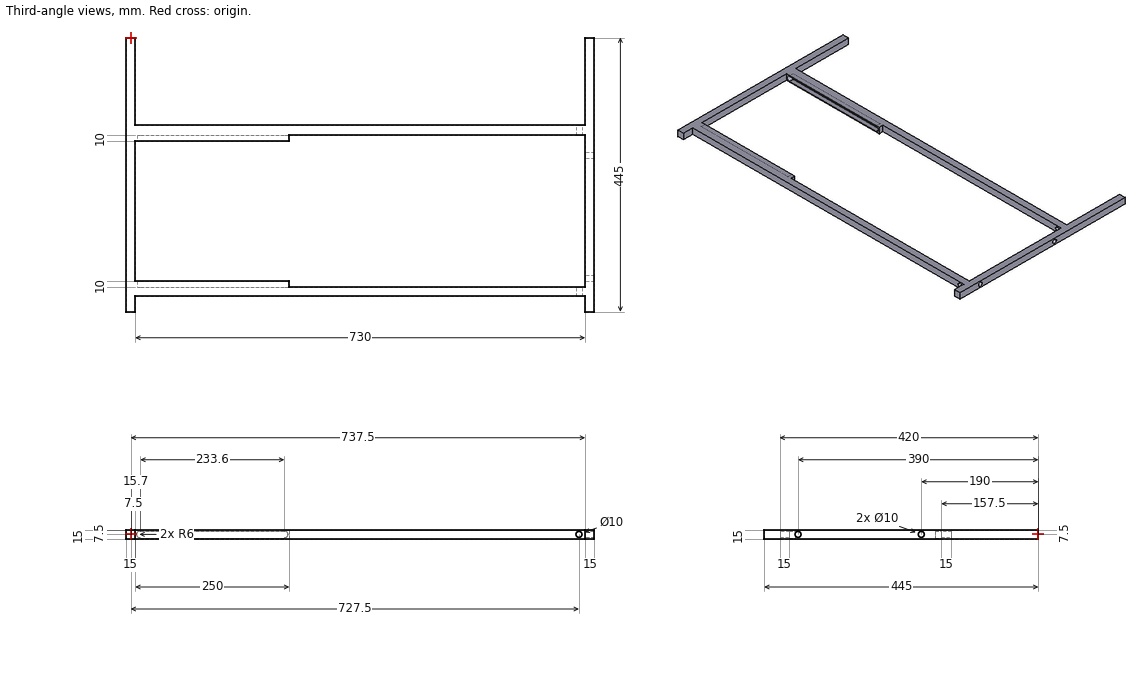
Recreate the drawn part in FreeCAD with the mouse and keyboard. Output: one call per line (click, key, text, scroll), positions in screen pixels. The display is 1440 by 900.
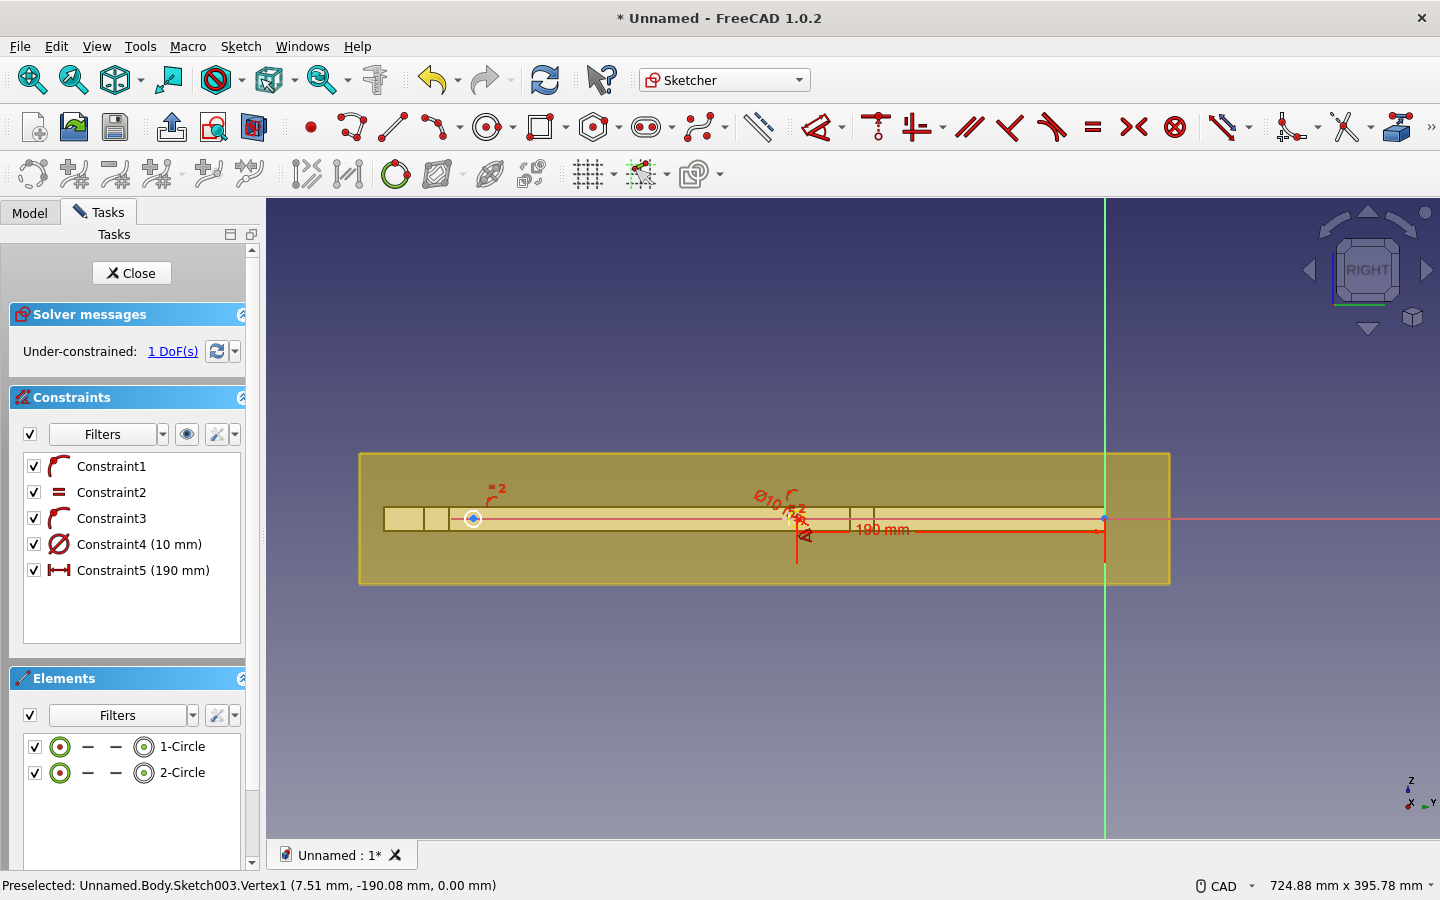
click(473, 519)
click(789, 553)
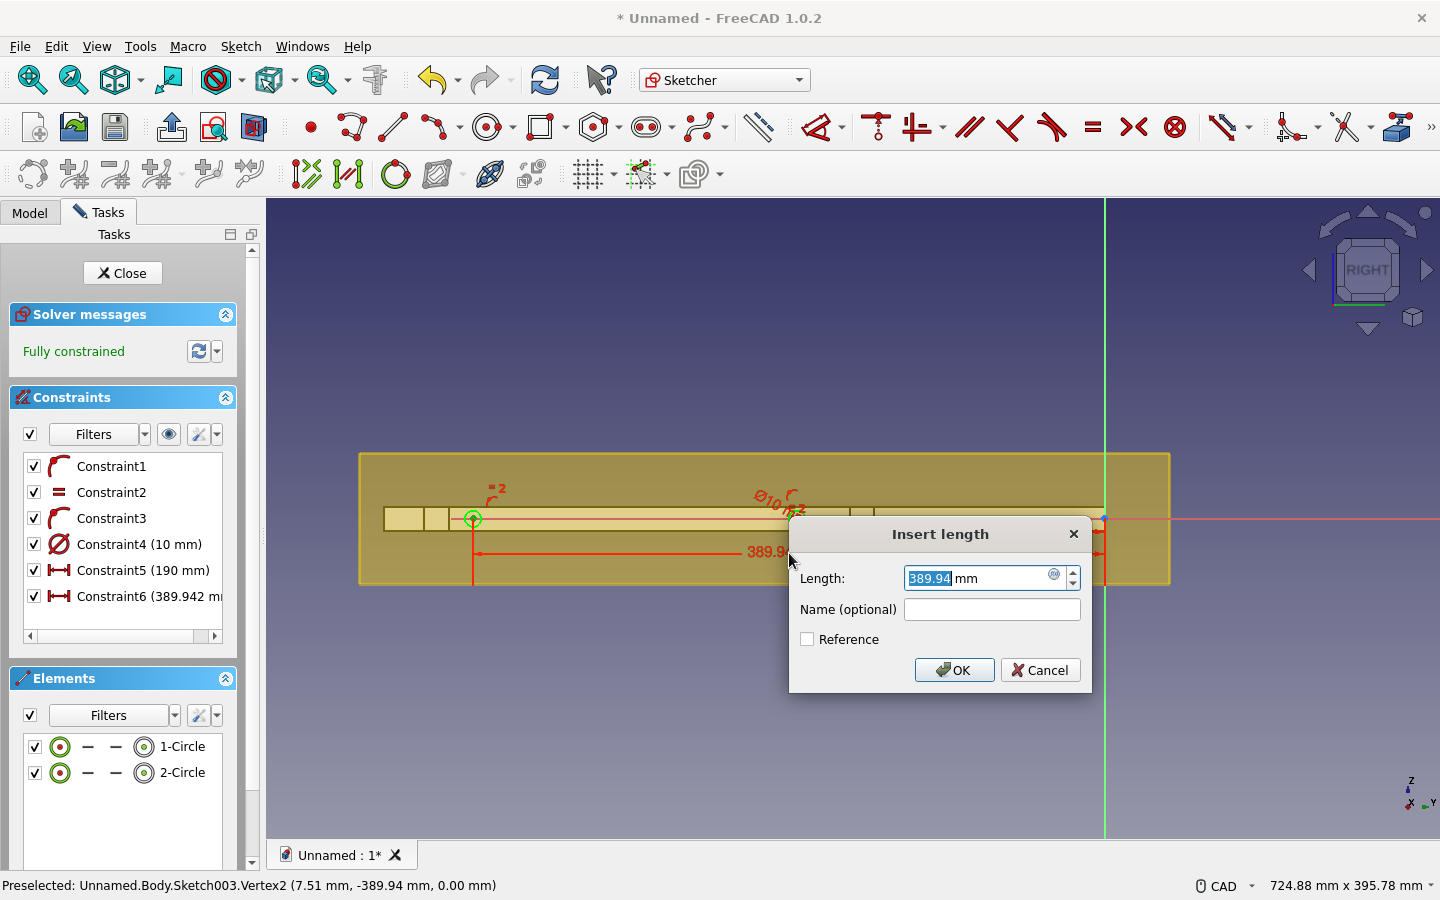
text(390)
key(Return)
key(Escape)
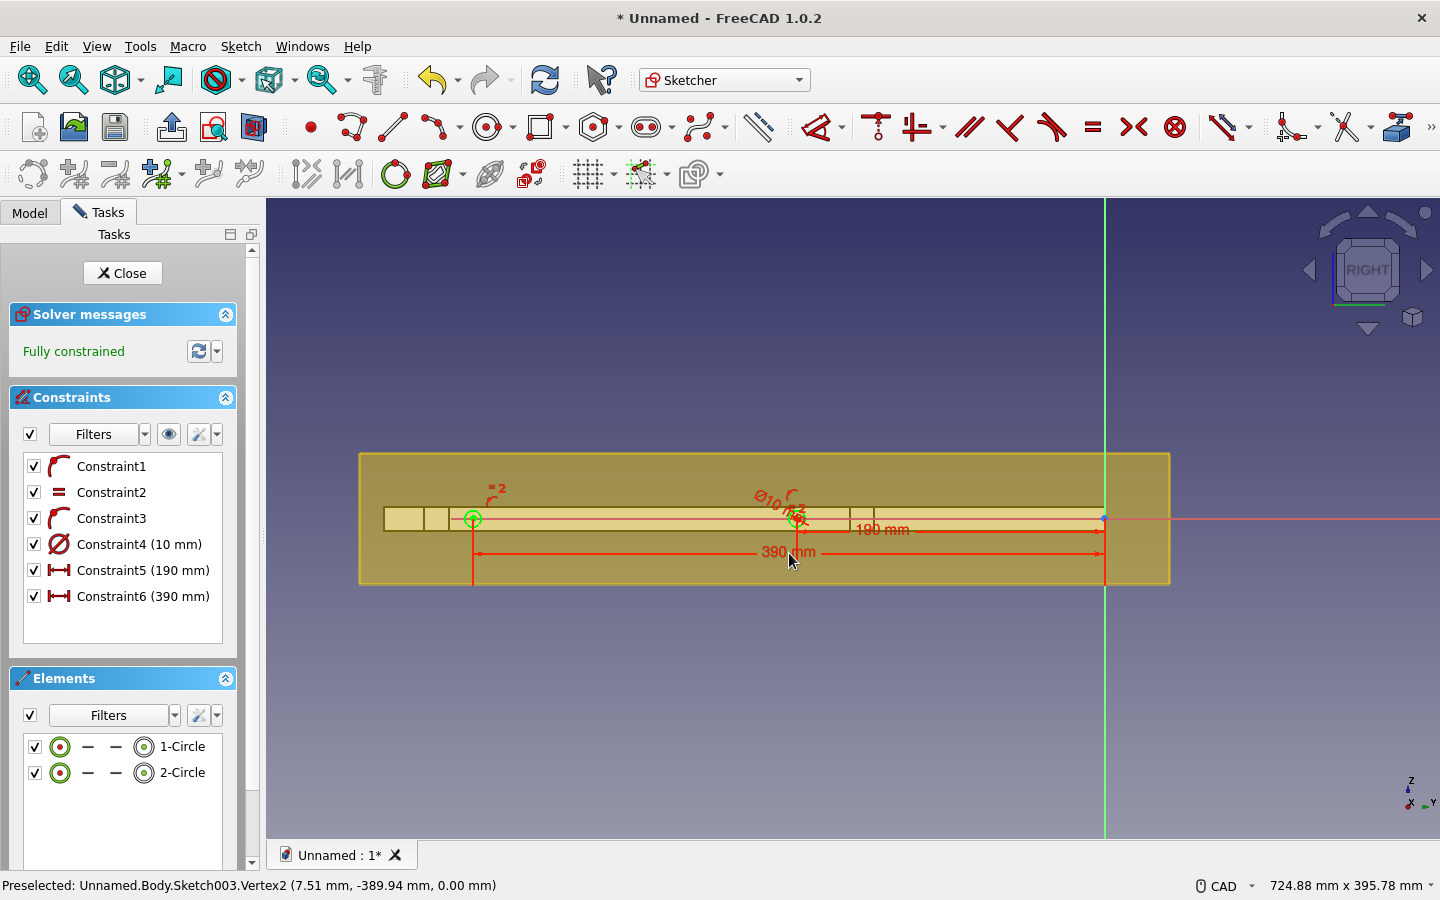
click(123, 273)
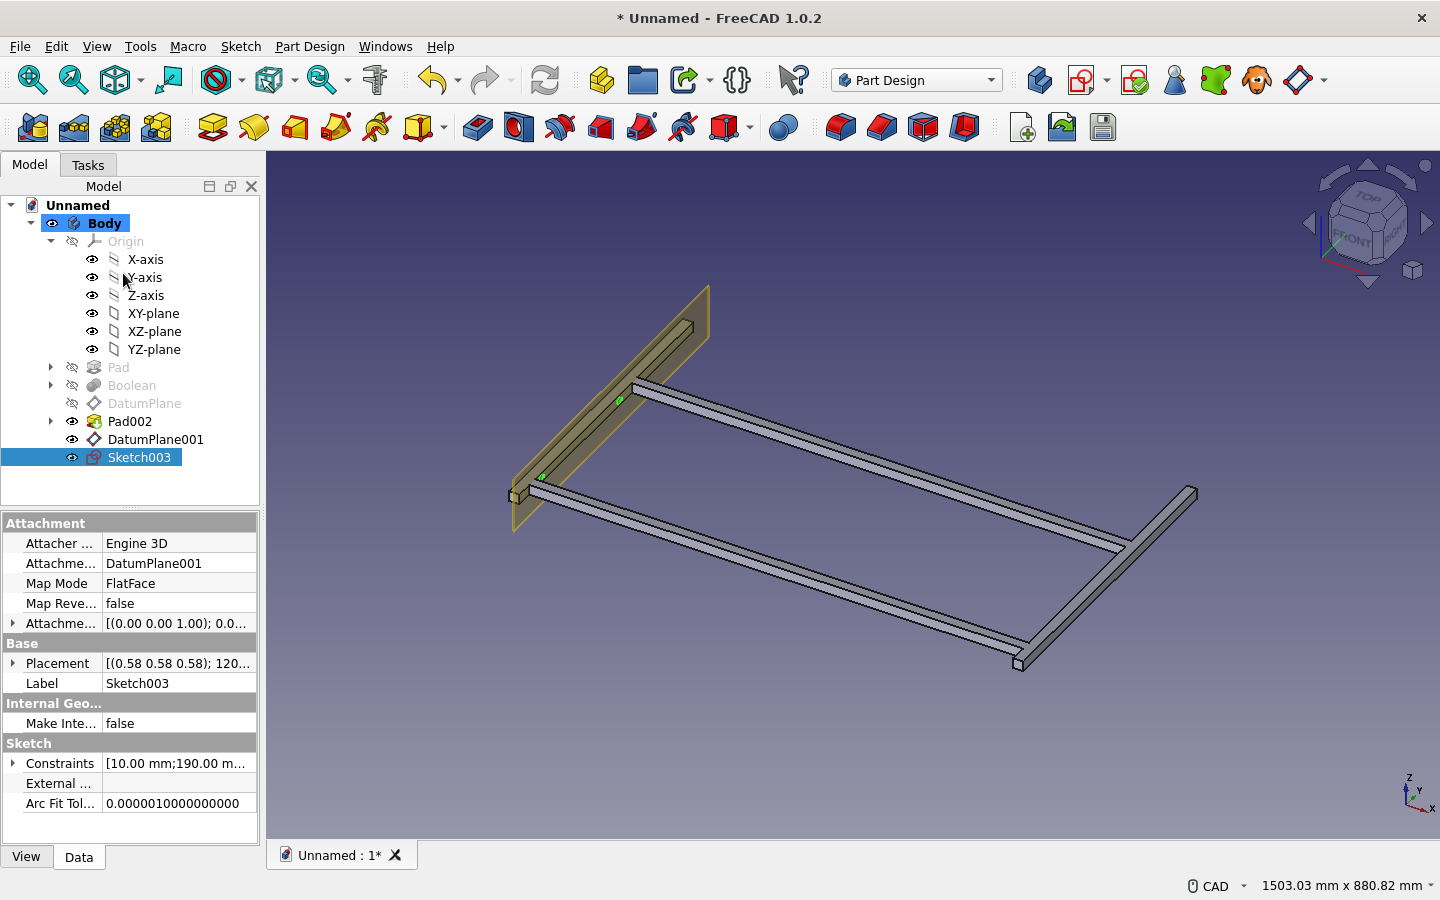
click(478, 128)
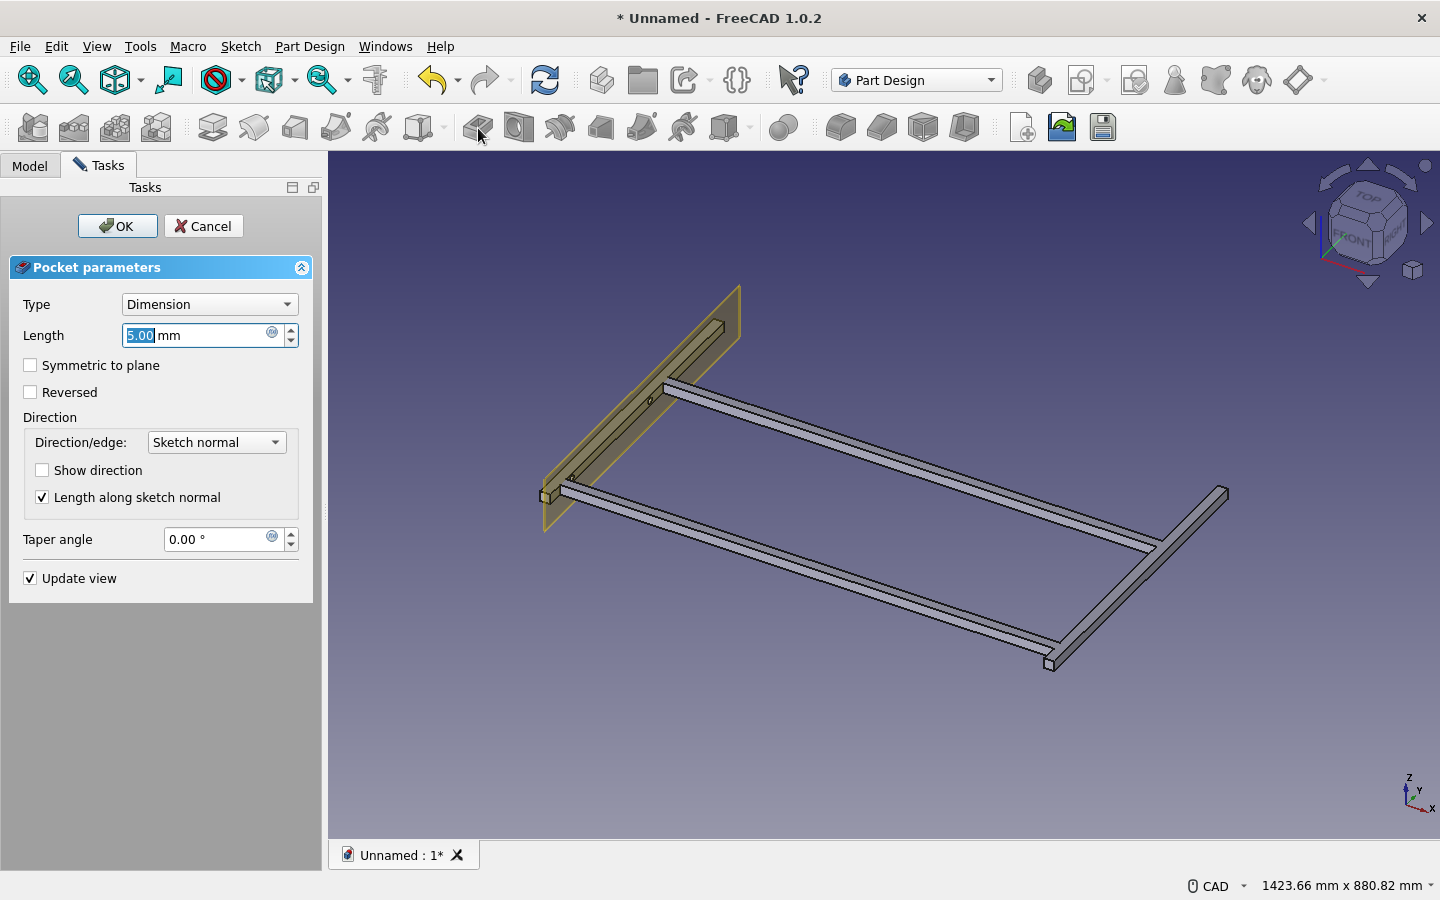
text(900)
key(Tab)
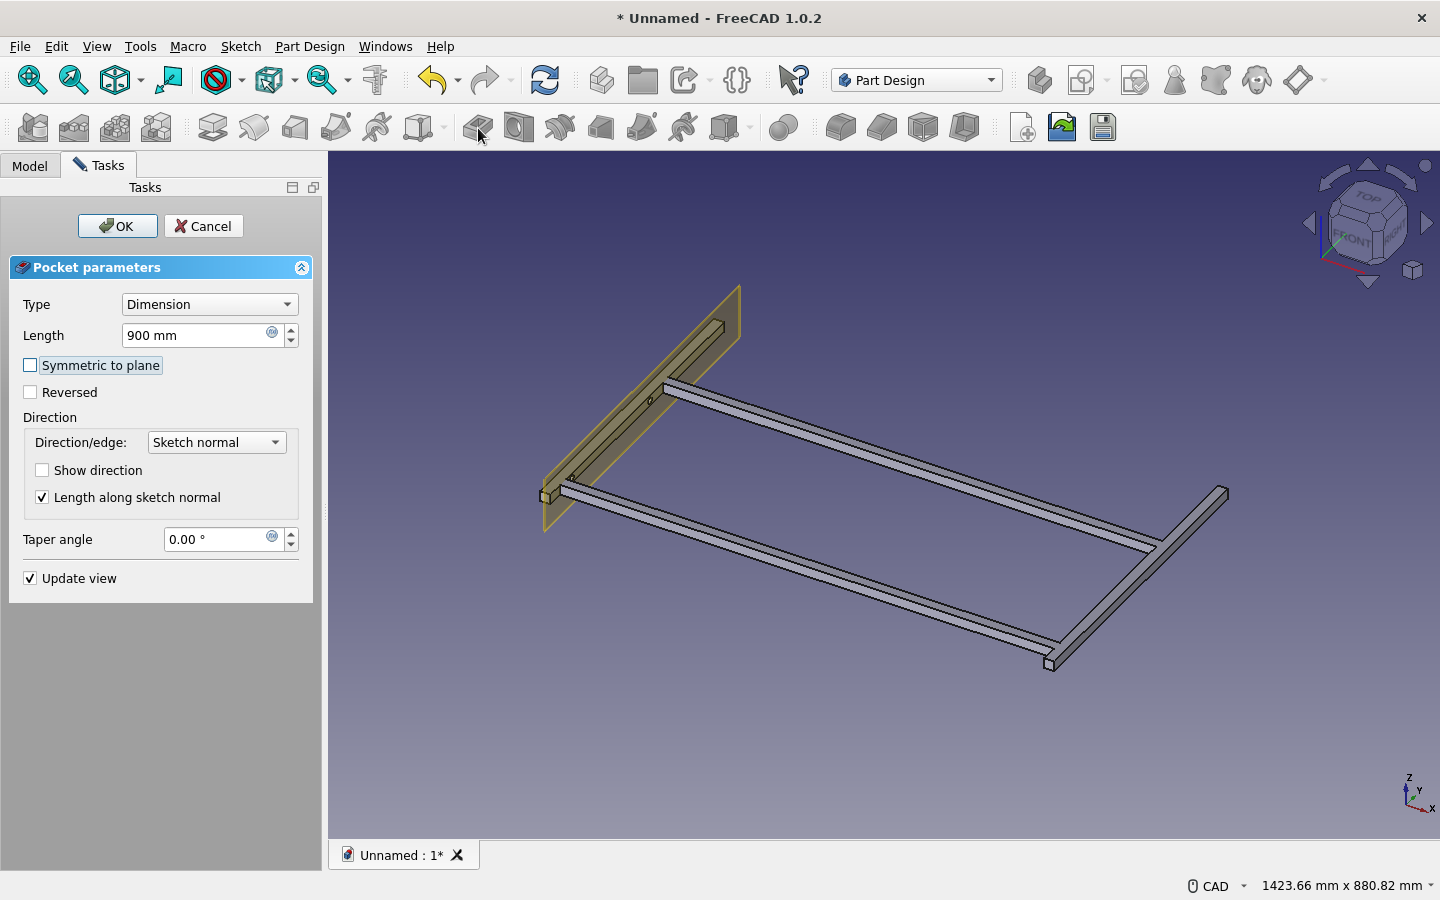
click(31, 392)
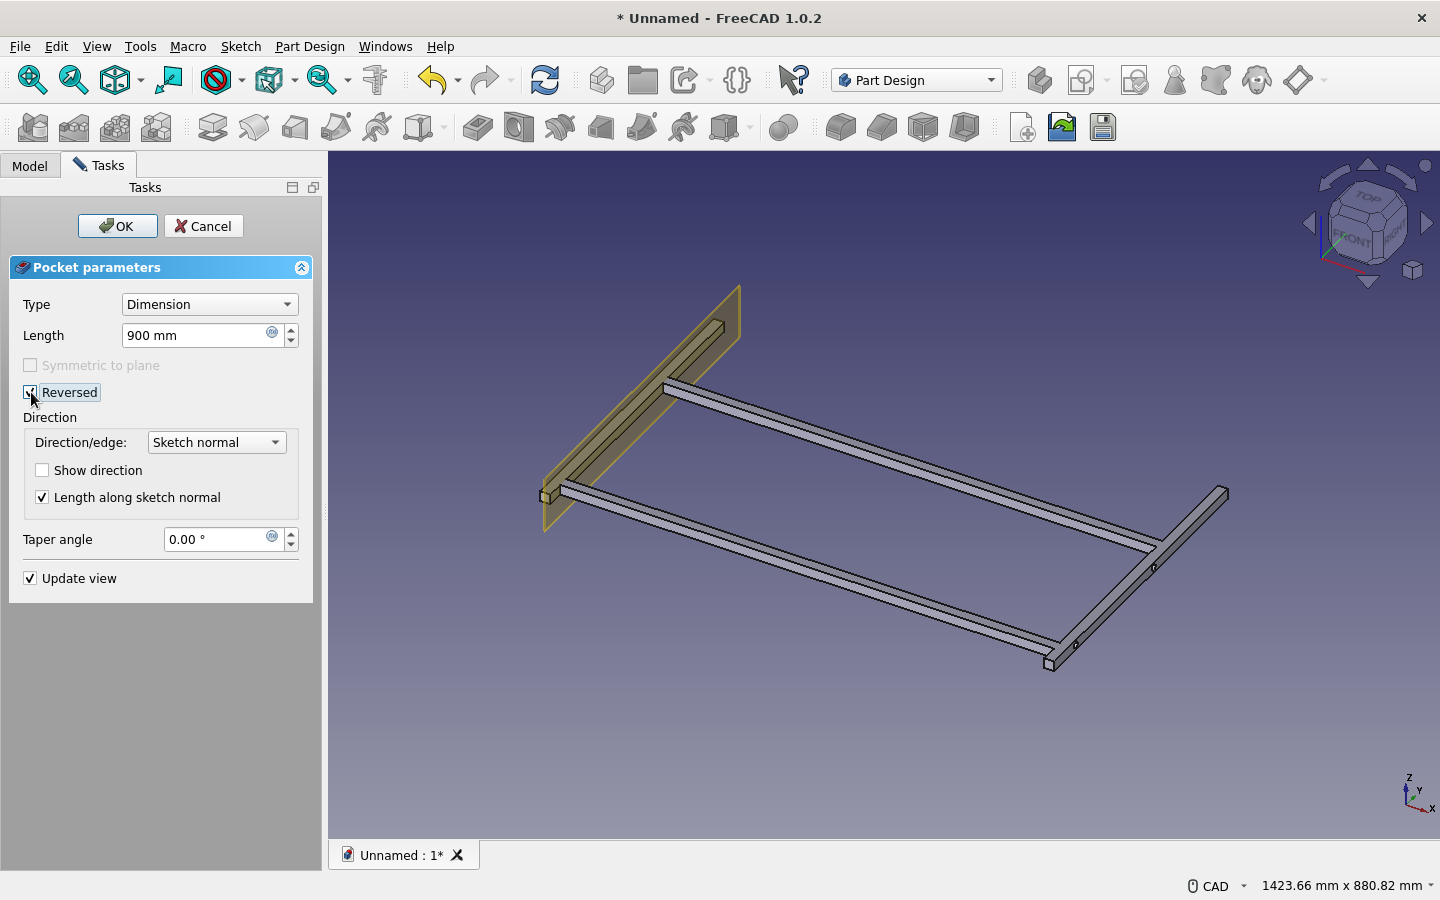
click(118, 226)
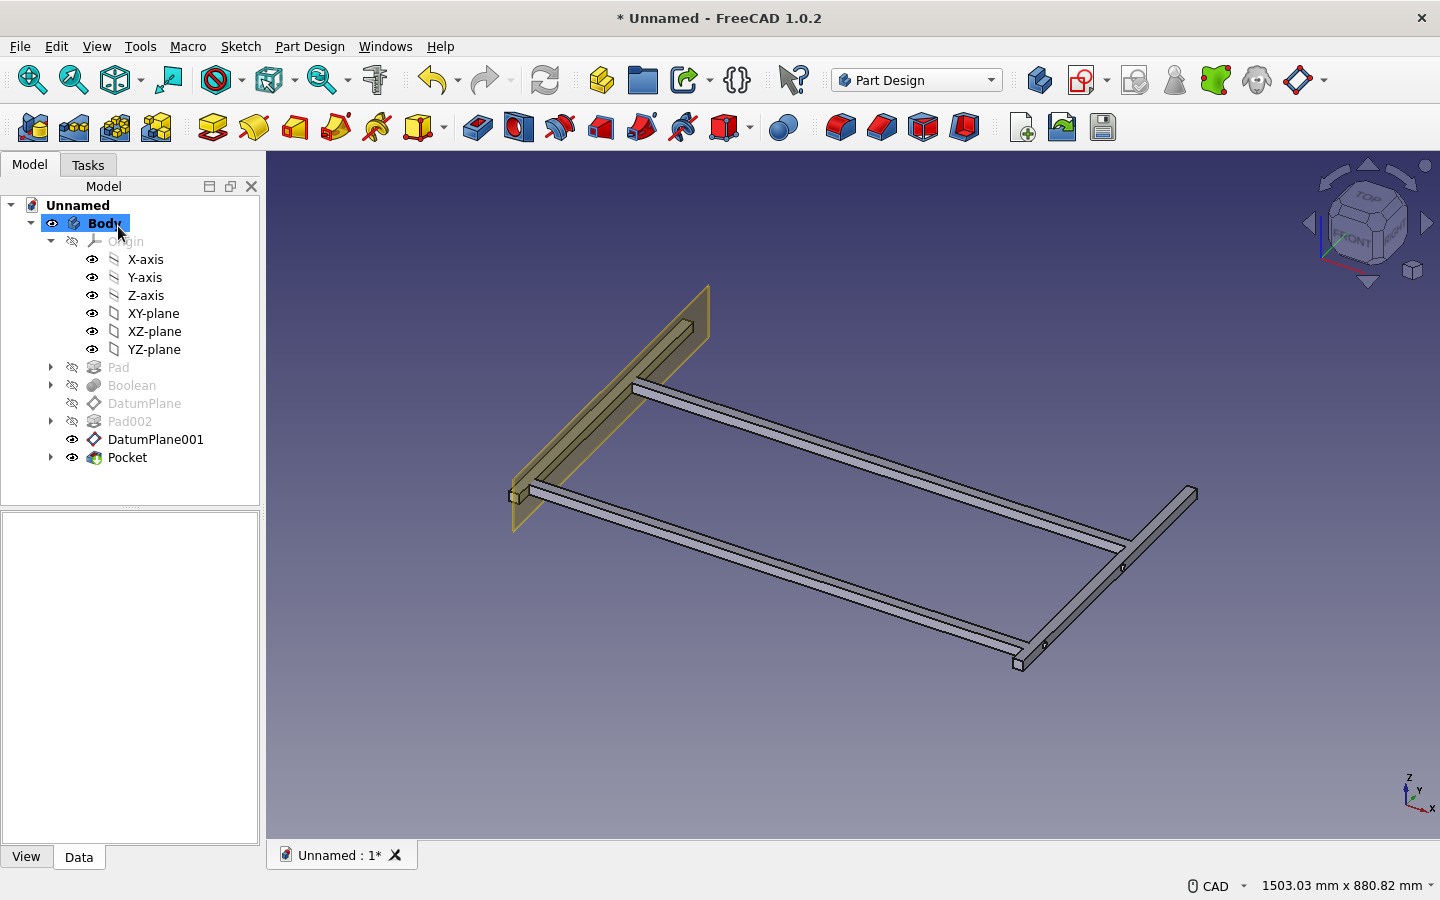
click(117, 439)
key(space)